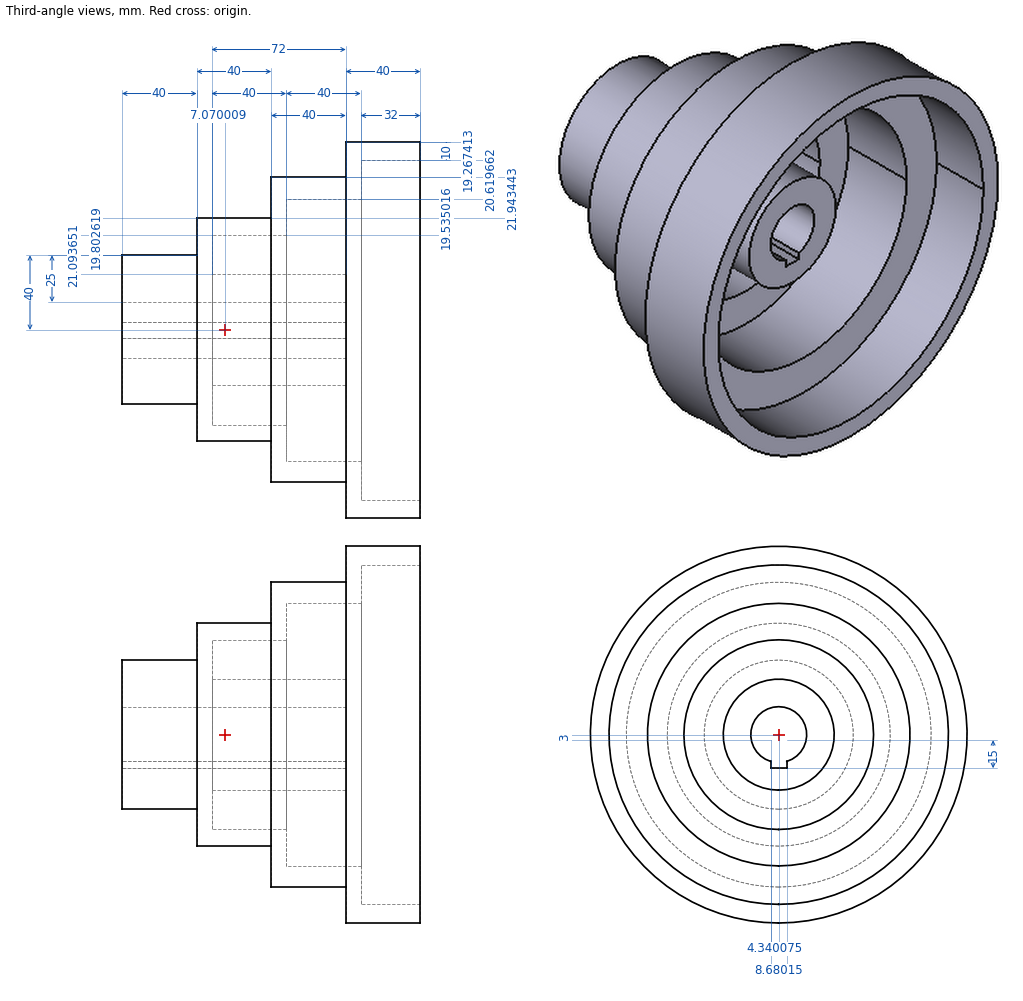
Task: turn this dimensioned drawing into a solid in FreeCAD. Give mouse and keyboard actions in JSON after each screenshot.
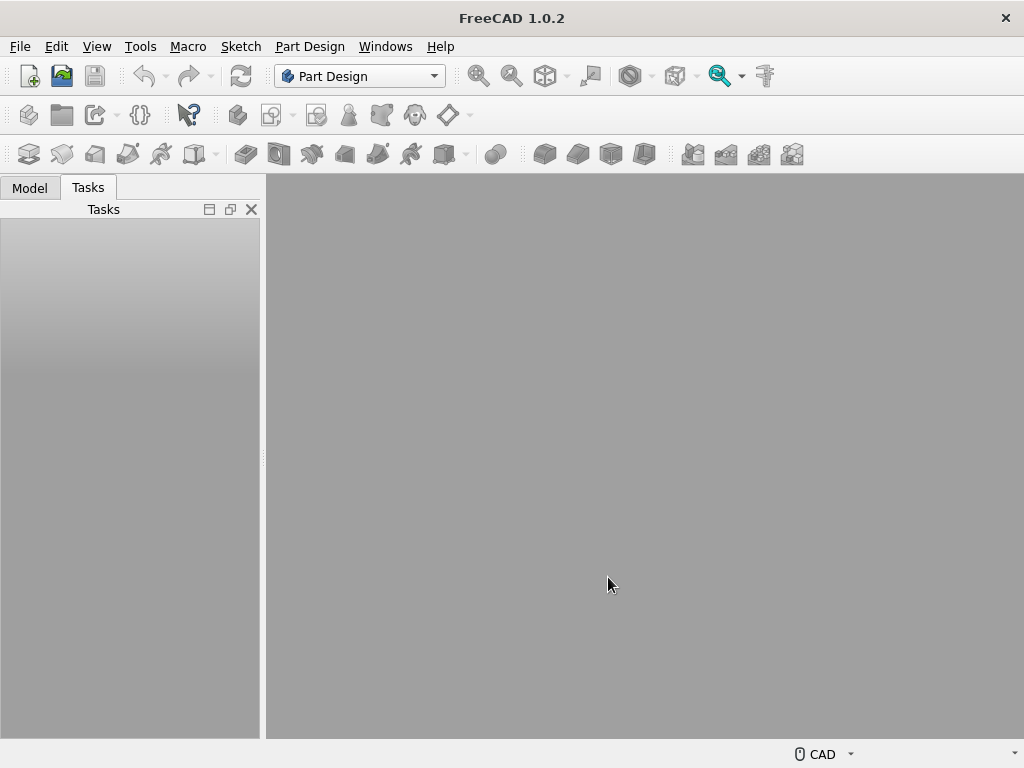
{"action": "left_click", "coordinate": [29, 76]}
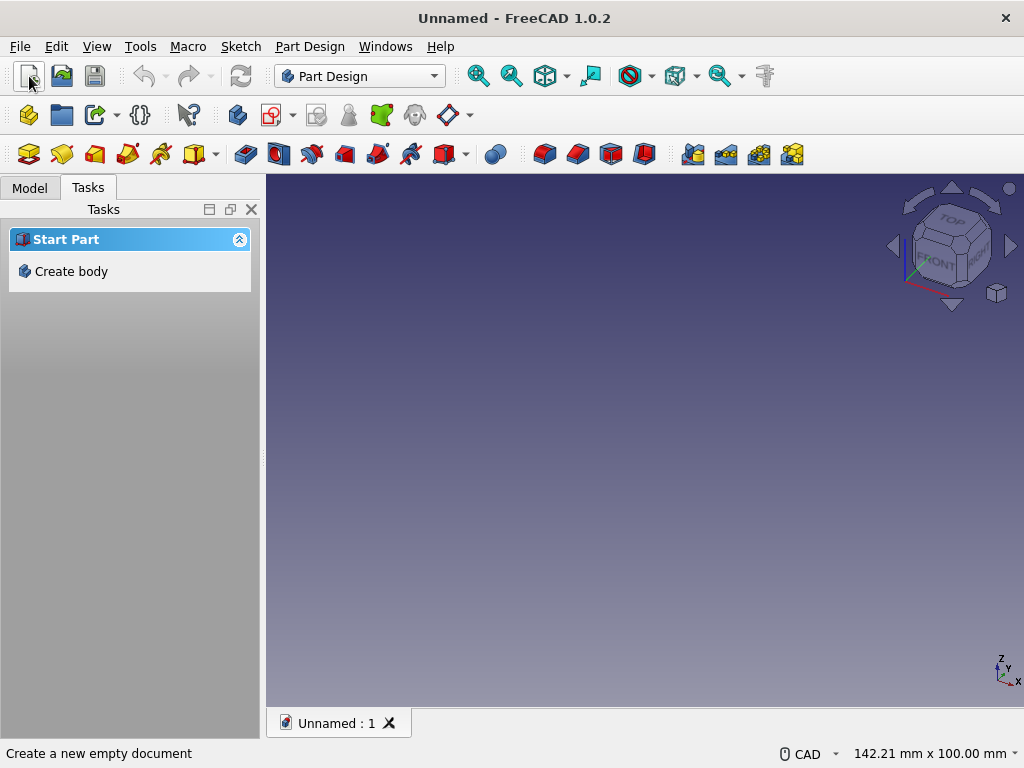
{"action": "left_click", "coordinate": [270, 116]}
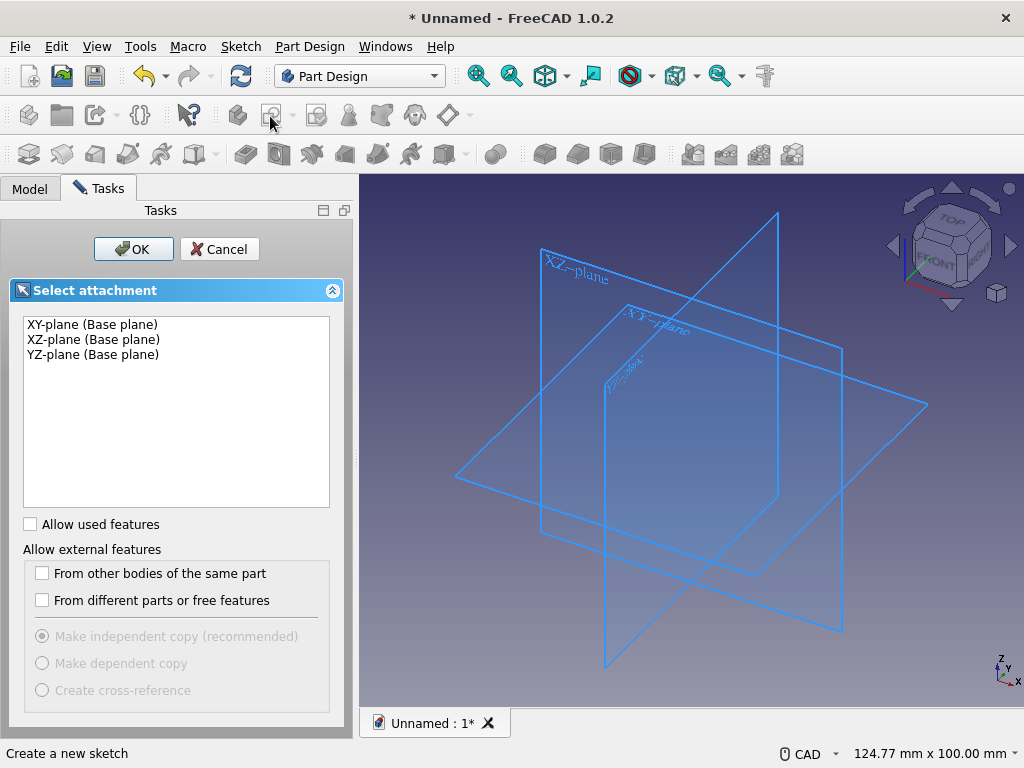
{"action": "left_click", "coordinate": [84, 324]}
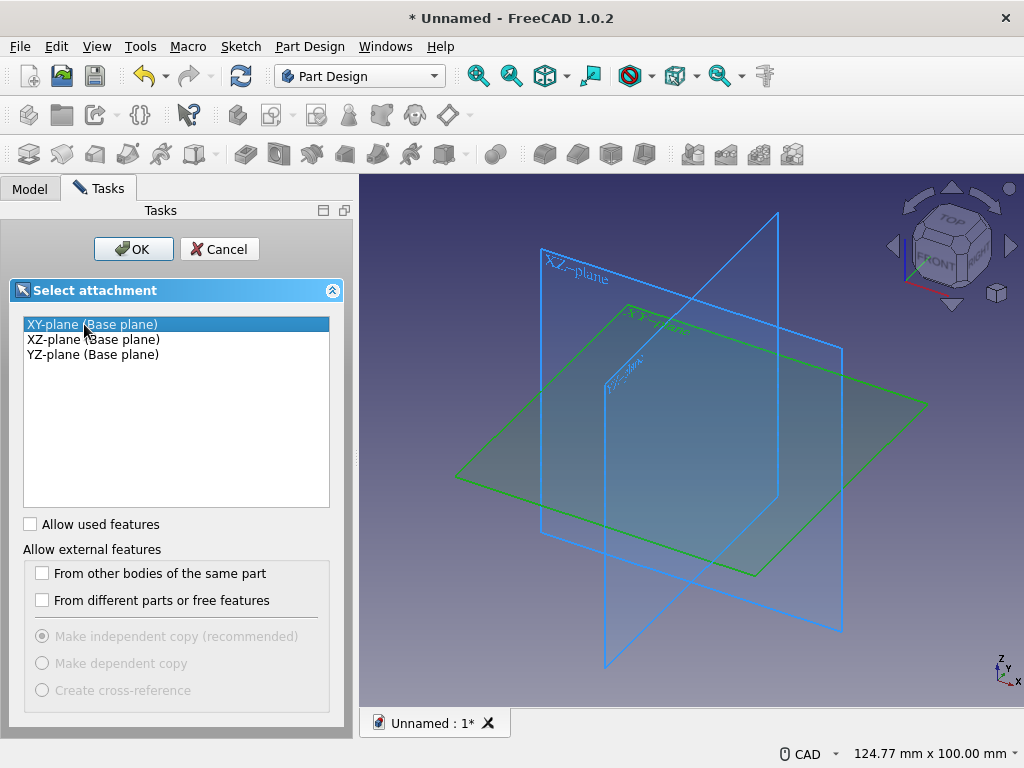
{"action": "left_click", "coordinate": [134, 249]}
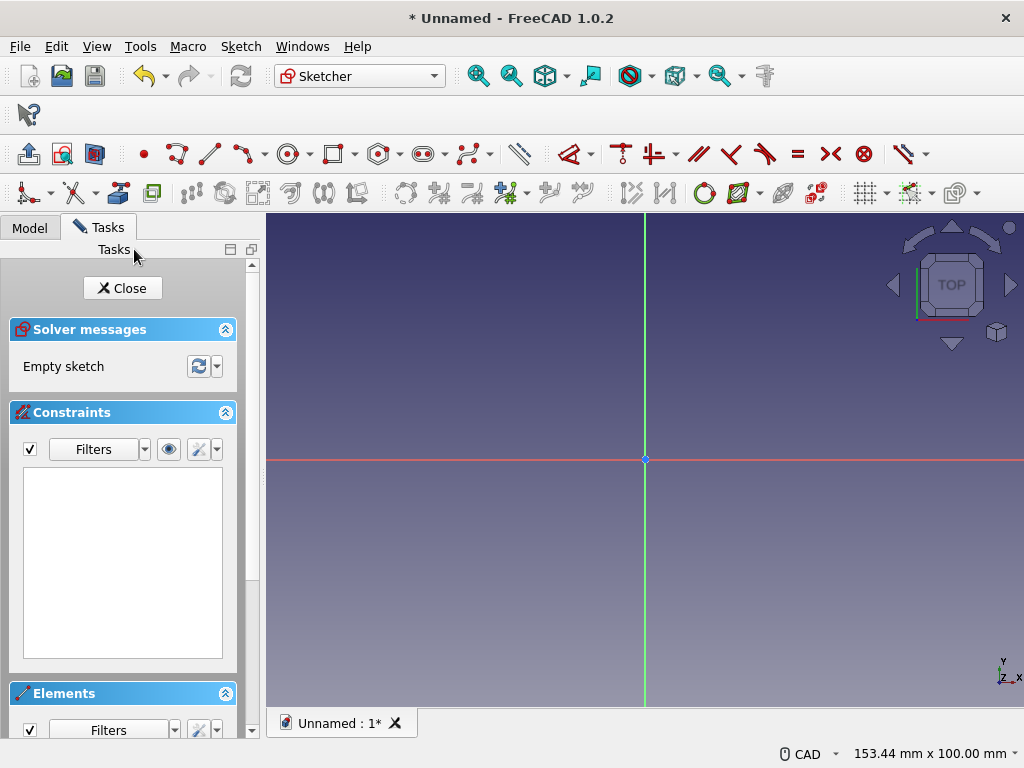
{"action": "scroll", "coordinate": [343, 679], "scroll_direction": "down", "scroll_amount": 3}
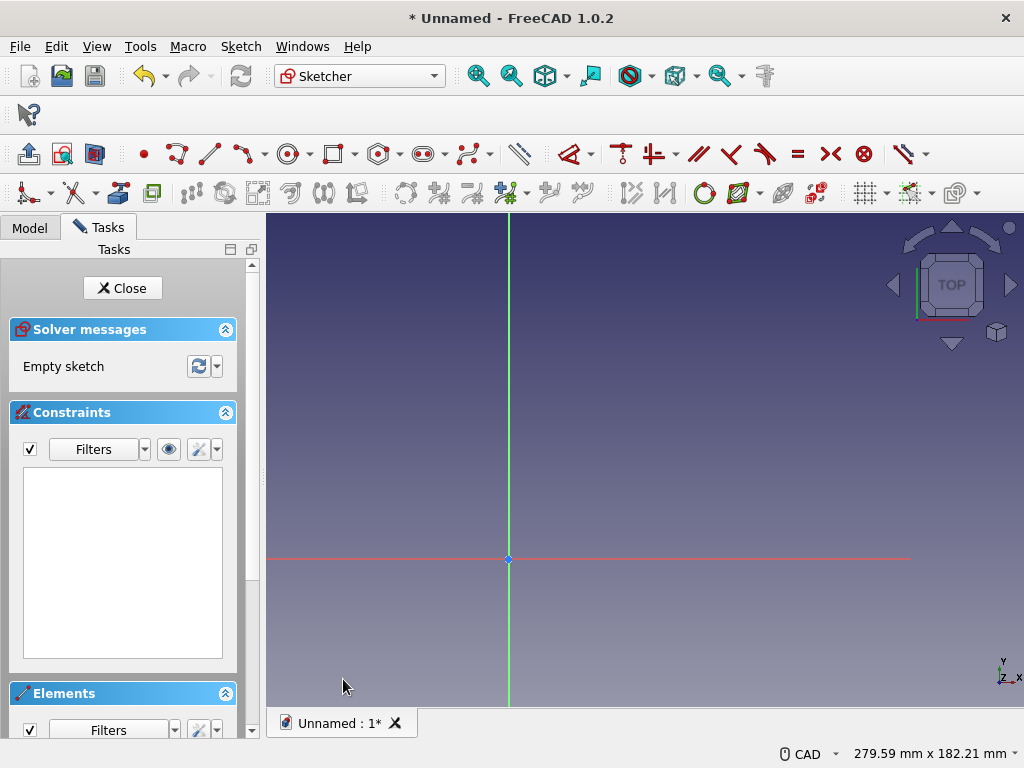
{"action": "left_click", "coordinate": [177, 154]}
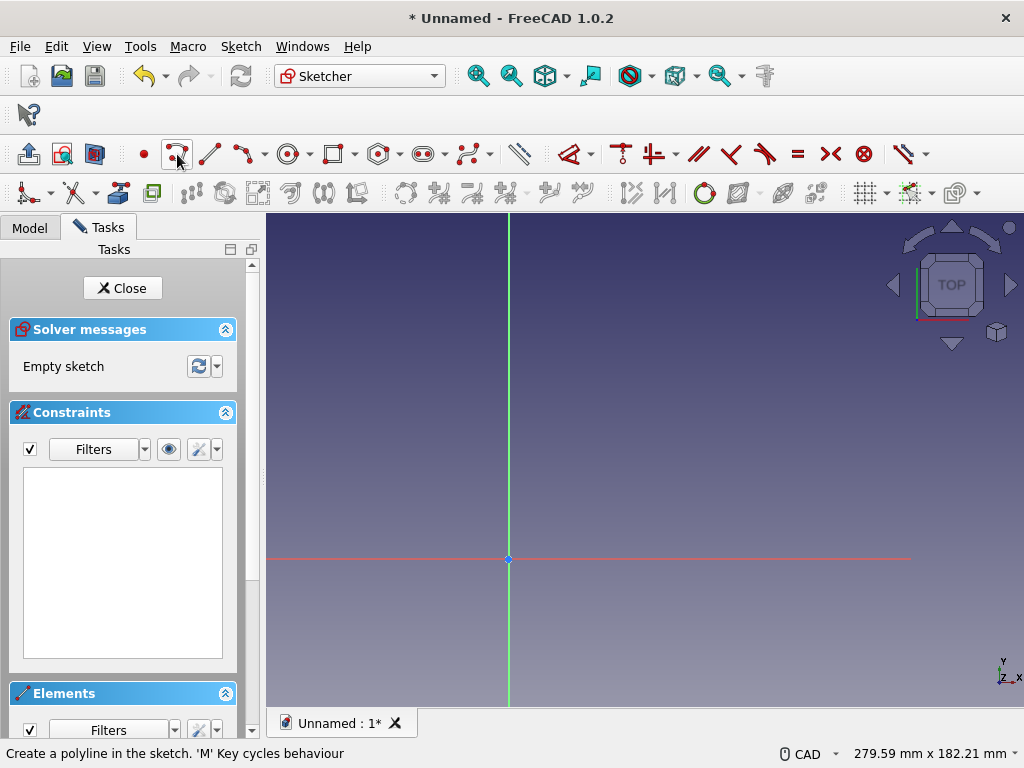
{"action": "left_click", "coordinate": [490, 479]}
{"action": "left_click", "coordinate": [490, 421]}
{"action": "left_click", "coordinate": [598, 421]}
{"action": "left_click", "coordinate": [598, 368]}
{"action": "left_click", "coordinate": [707, 368]}
{"action": "left_click", "coordinate": [707, 312]}
{"action": "left_click", "coordinate": [793, 312]}
{"action": "left_click", "coordinate": [793, 285]}
{"action": "left_click", "coordinate": [685, 285]}
{"action": "left_click", "coordinate": [685, 338]}
{"action": "left_click", "coordinate": [576, 338]}
{"action": "left_click", "coordinate": [576, 397]}
{"action": "left_click", "coordinate": [468, 397]}
{"action": "left_click", "coordinate": [468, 451]}
{"action": "left_click", "coordinate": [359, 451]}
{"action": "left_click", "coordinate": [359, 519]}
{"action": "left_click", "coordinate": [685, 519]}
{"action": "left_click", "coordinate": [685, 479]}
{"action": "left_click", "coordinate": [490, 480]}
{"action": "key", "text": "Escape"}
{"action": "key", "text": "Escape"}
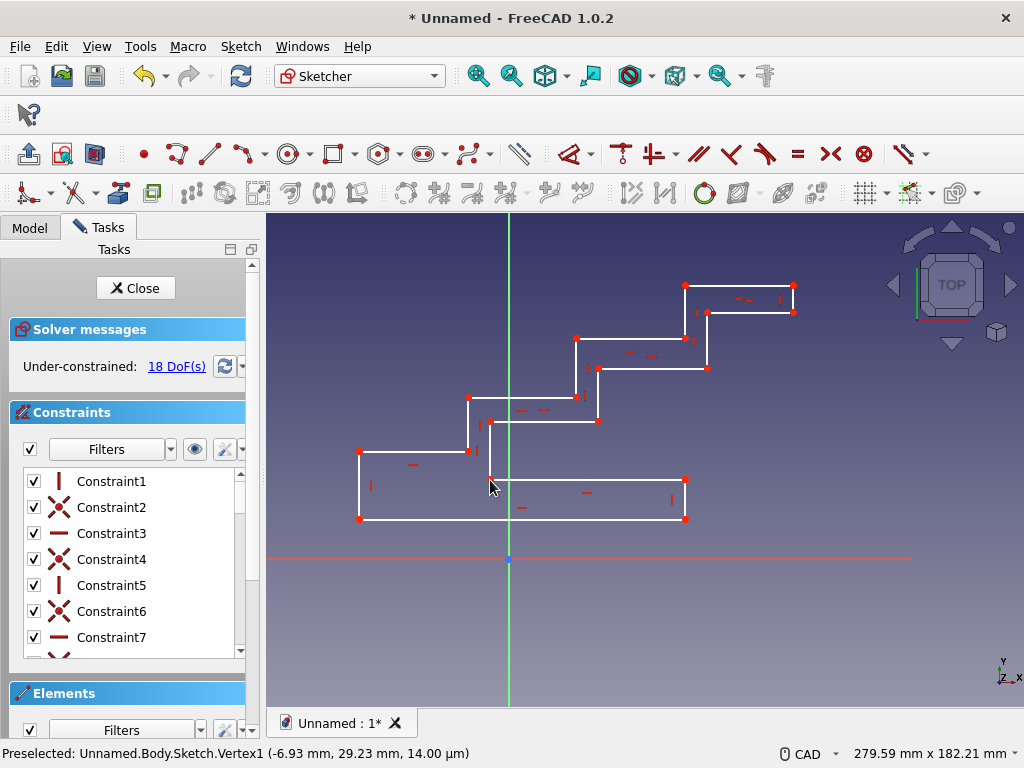
{"action": "left_click", "coordinate": [522, 422]}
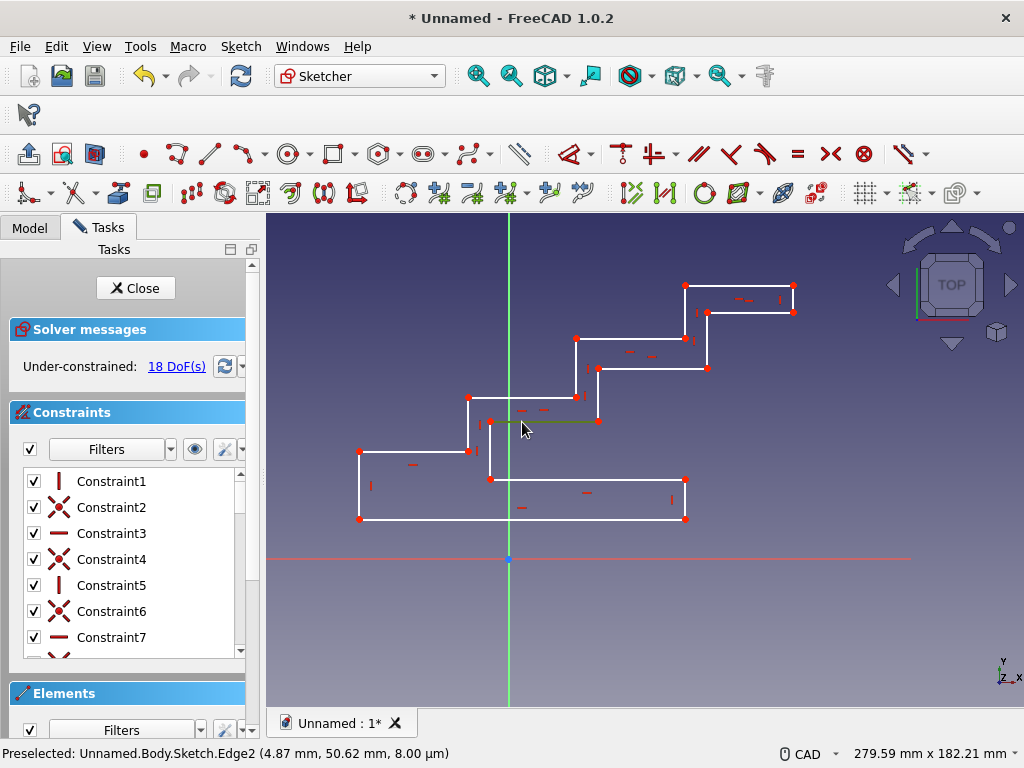
{"action": "left_click", "coordinate": [590, 154]}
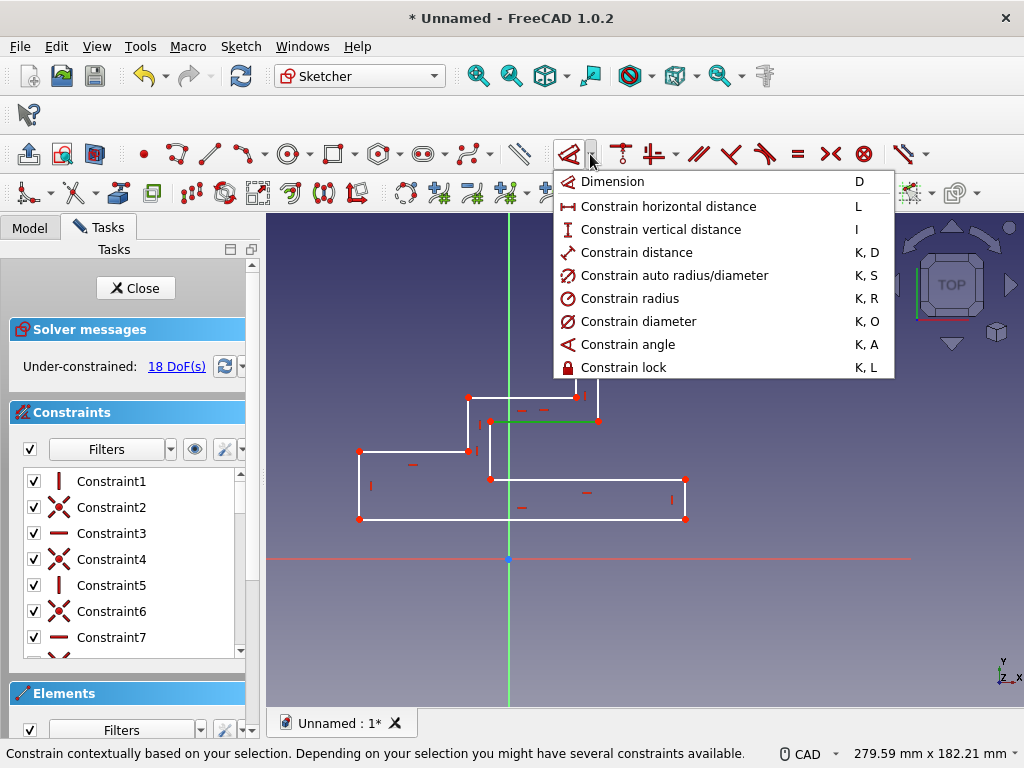
{"action": "left_click", "coordinate": [724, 206]}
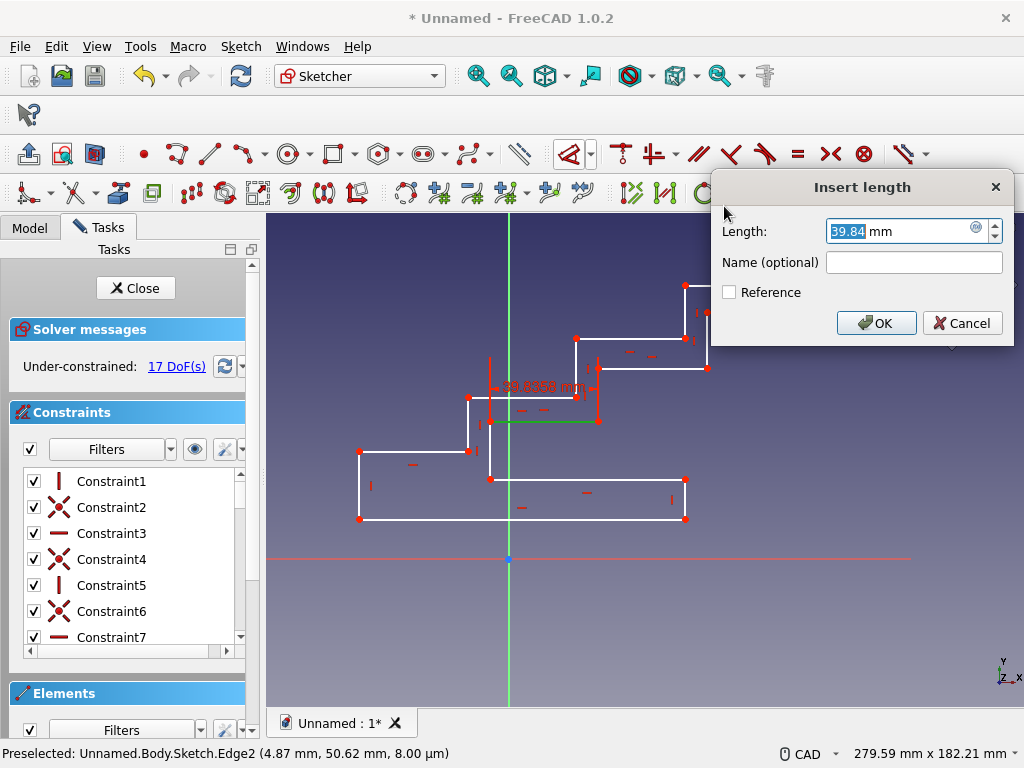
{"action": "type", "text": "40"}
{"action": "key", "text": "Return"}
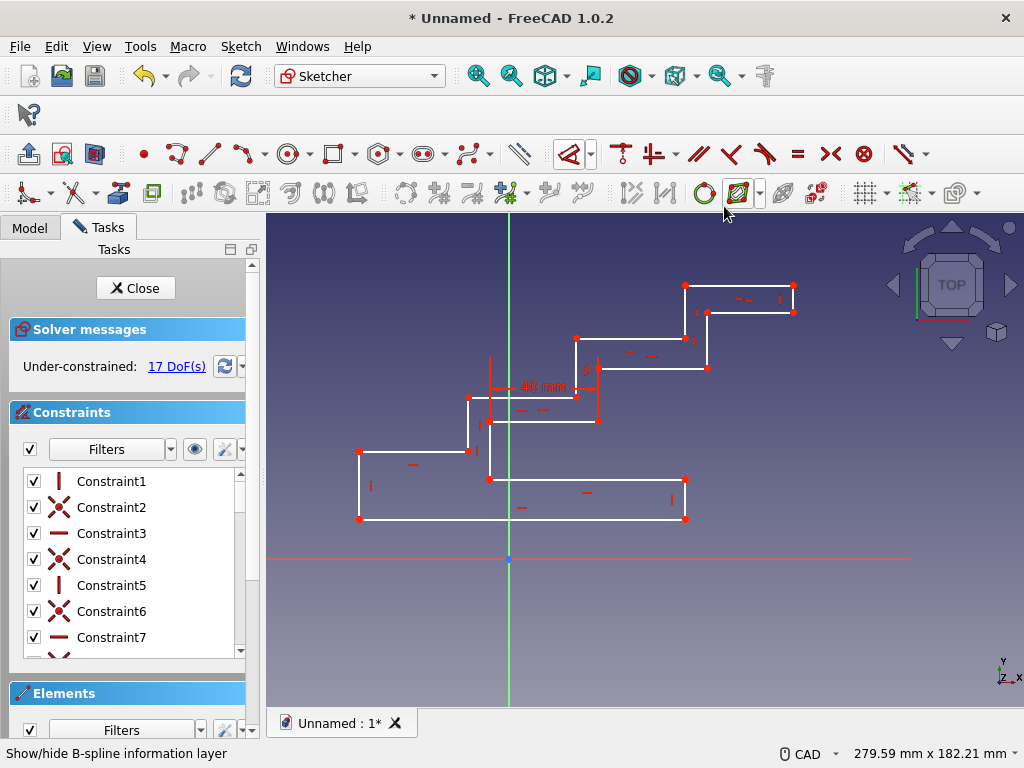
{"action": "left_click", "coordinate": [631, 369]}